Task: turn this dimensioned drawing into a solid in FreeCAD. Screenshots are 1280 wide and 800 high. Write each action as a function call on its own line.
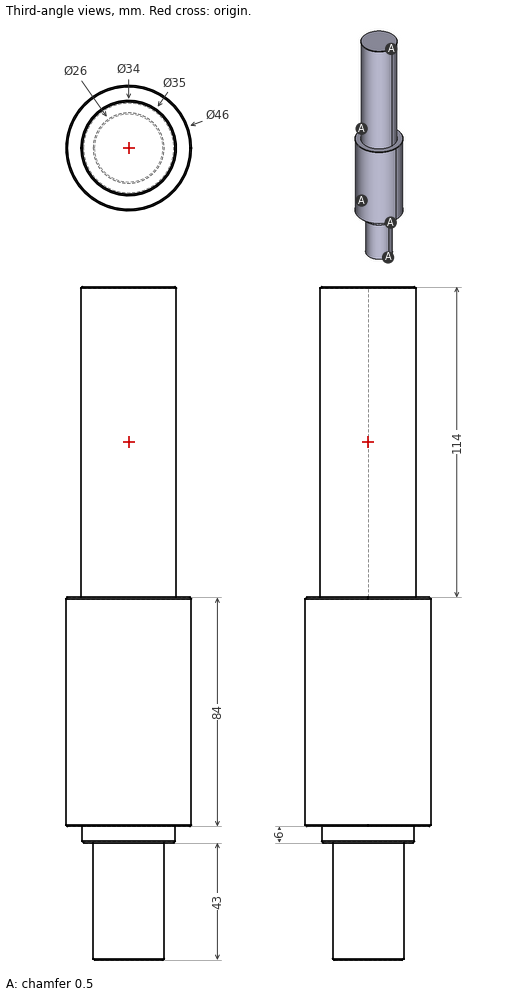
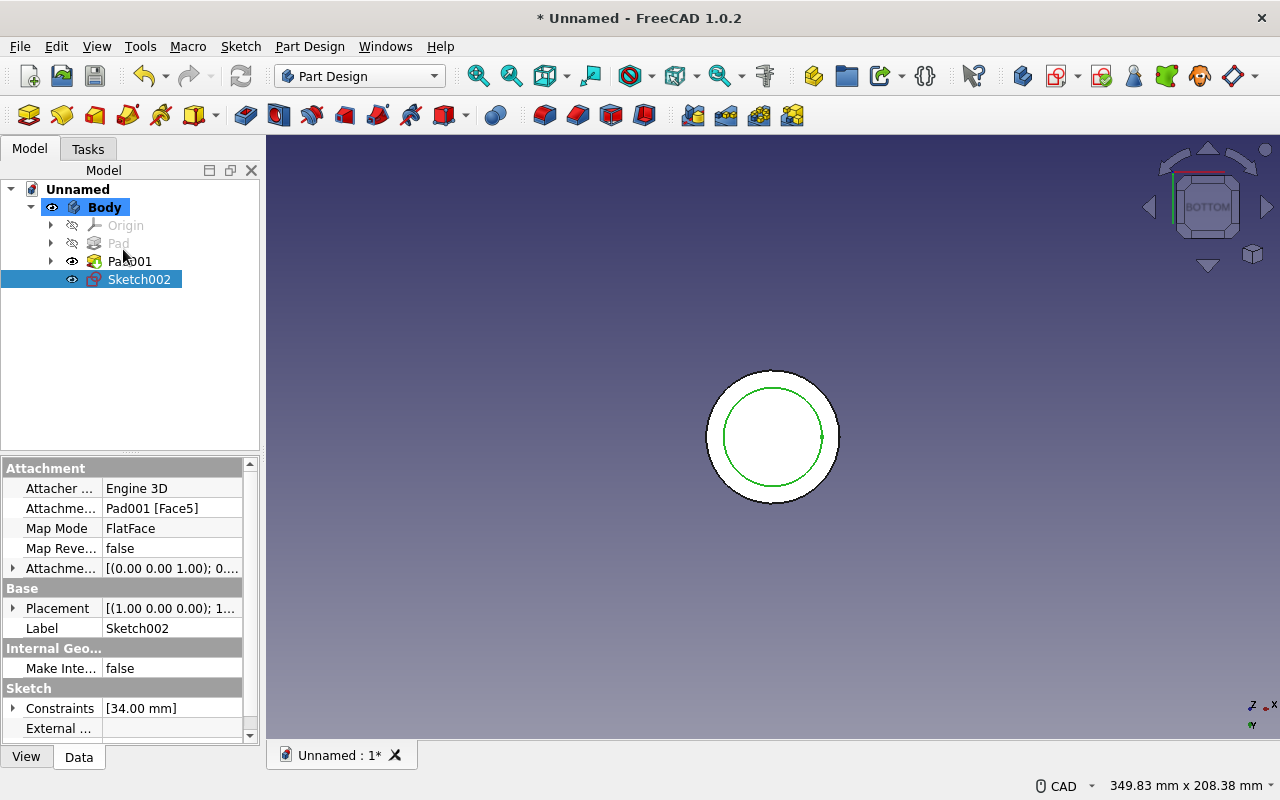
click(29, 116)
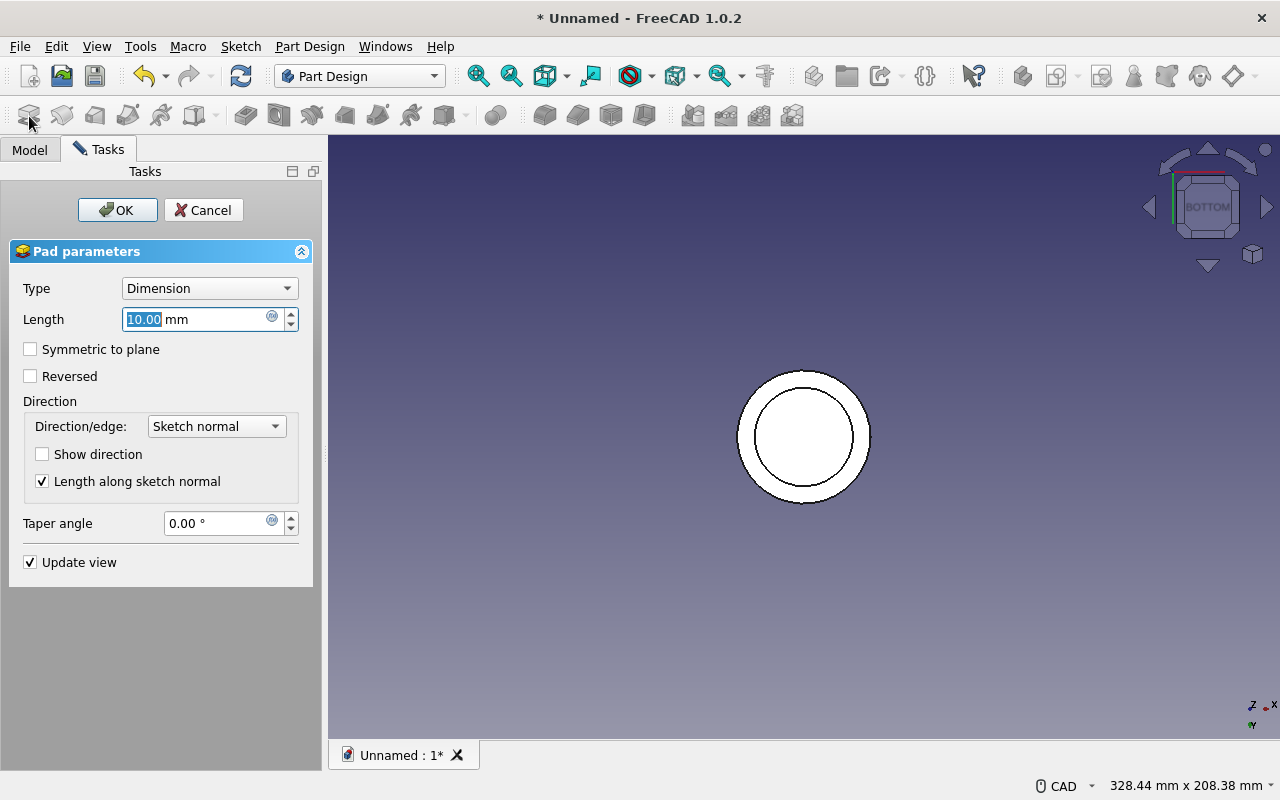
text(6)
key(Tab)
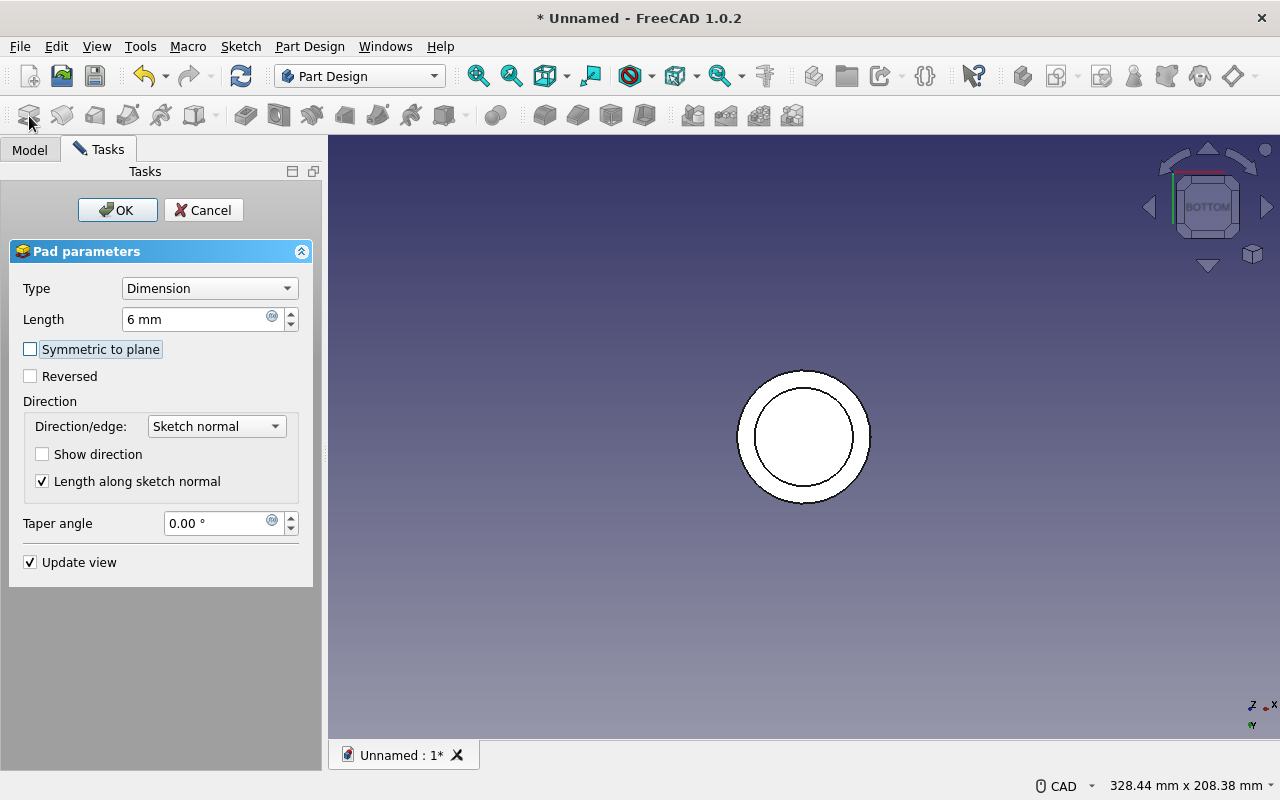
click(118, 210)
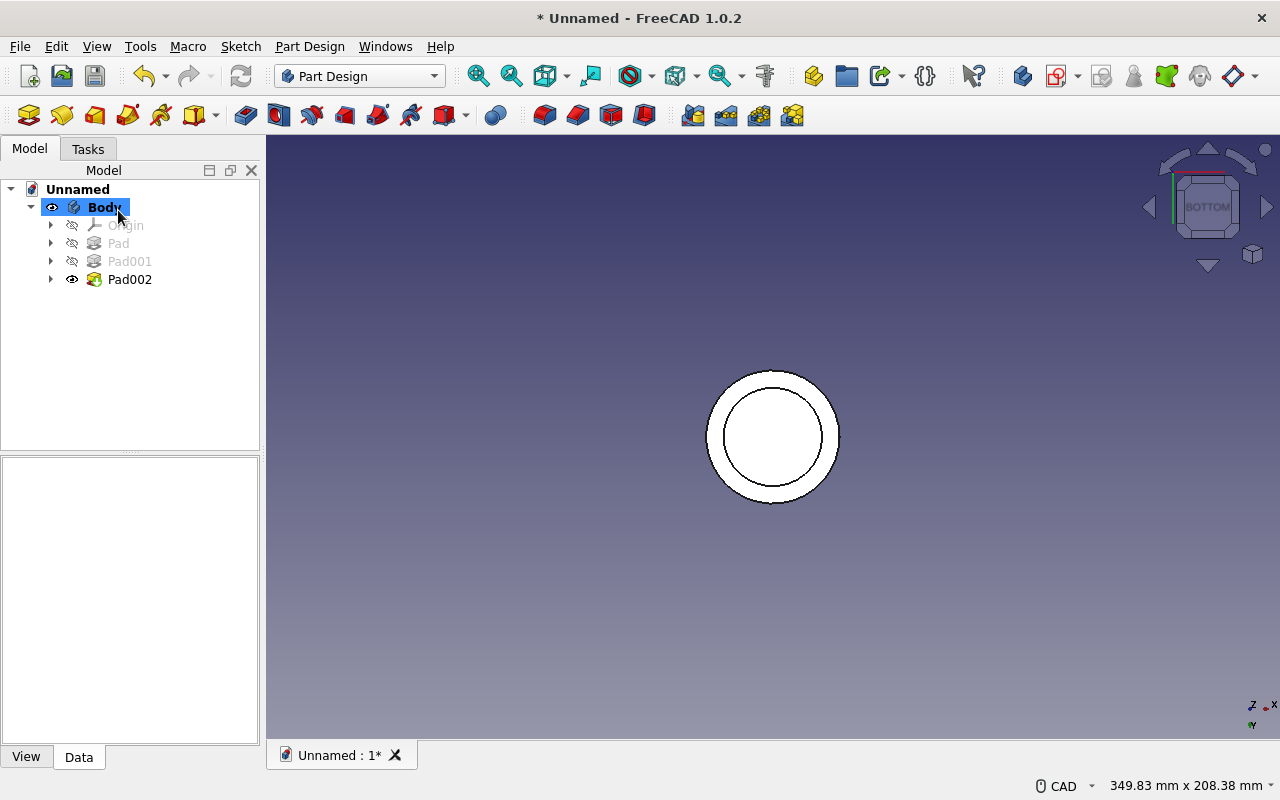
key(v)
key(f)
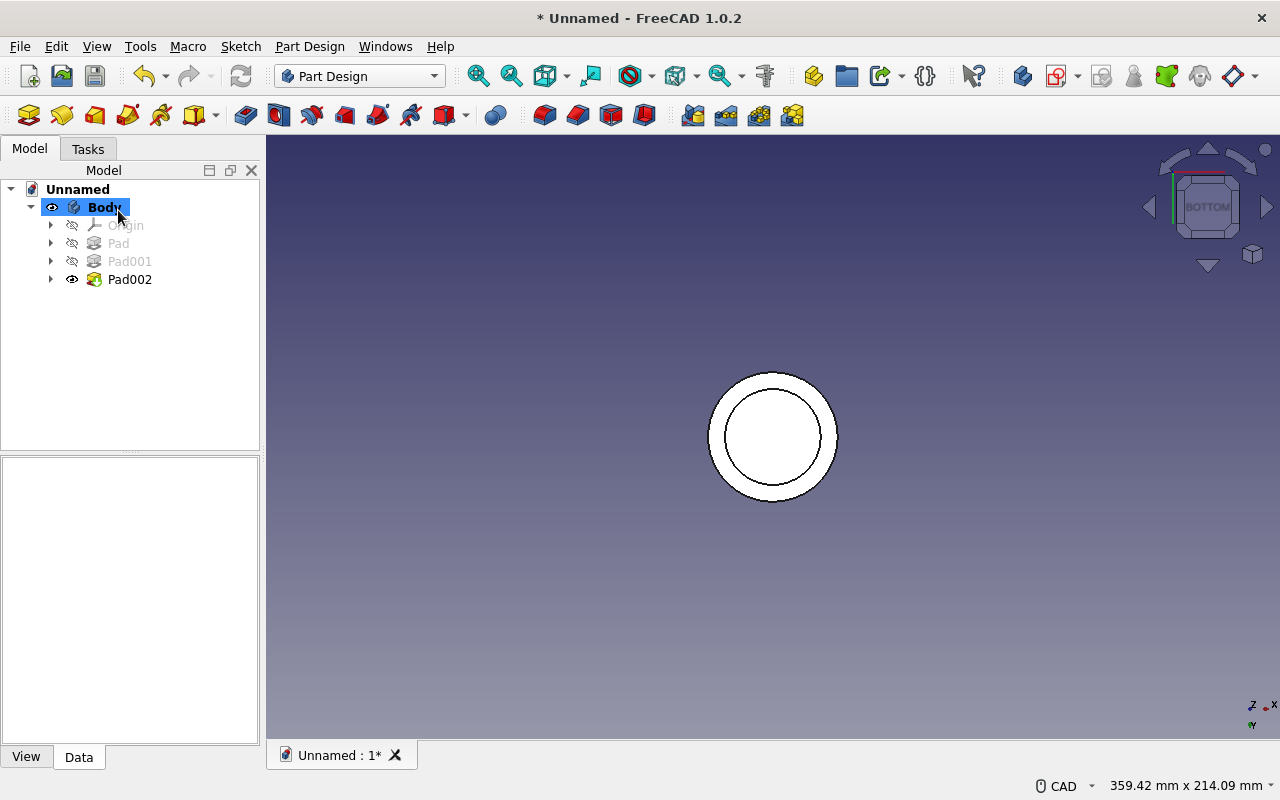
click(773, 436)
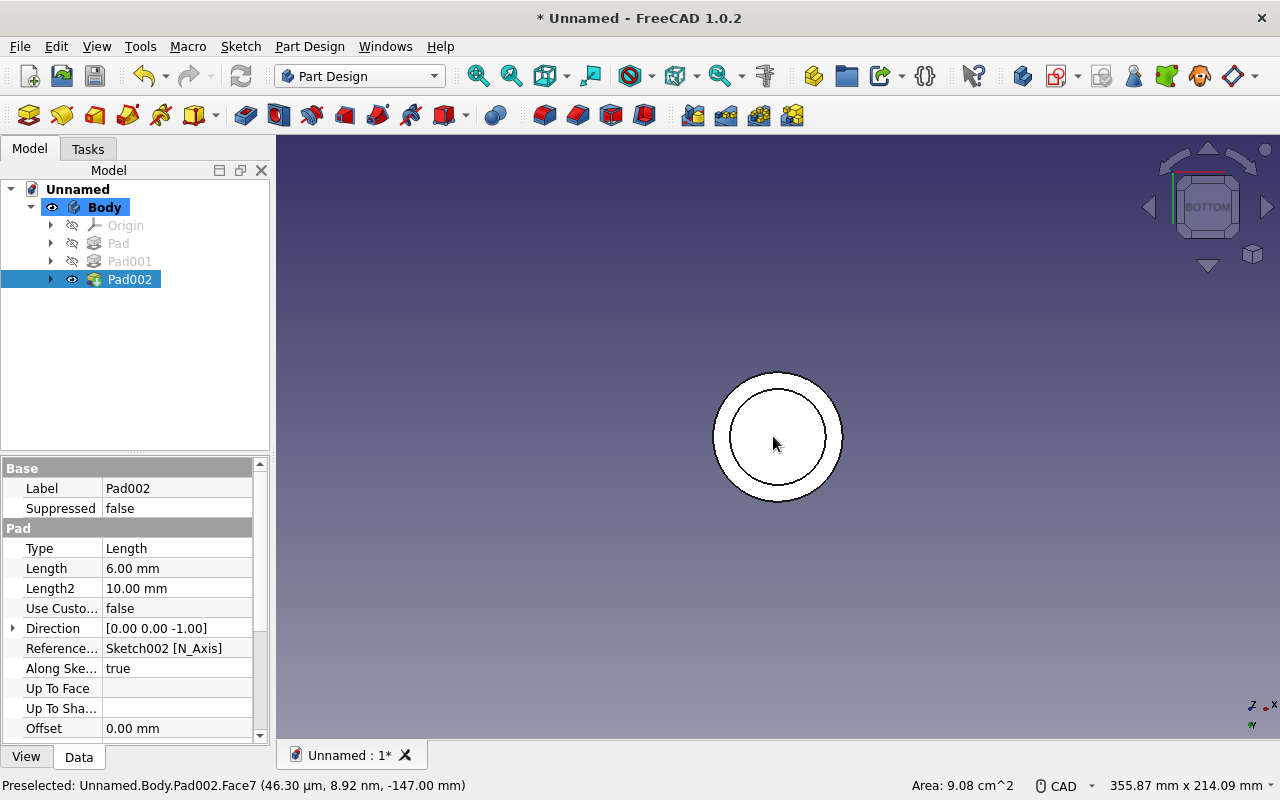
click(1056, 76)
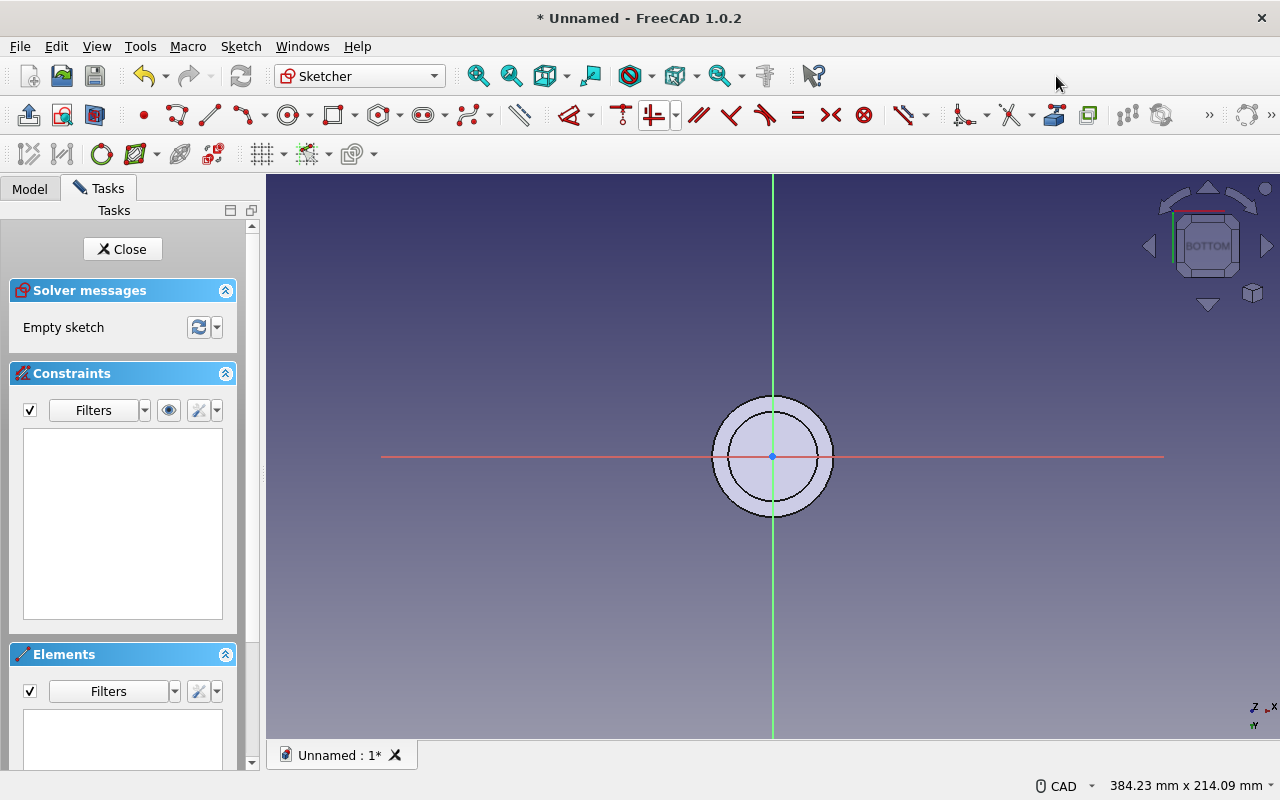
scroll(790, 456, up, 8)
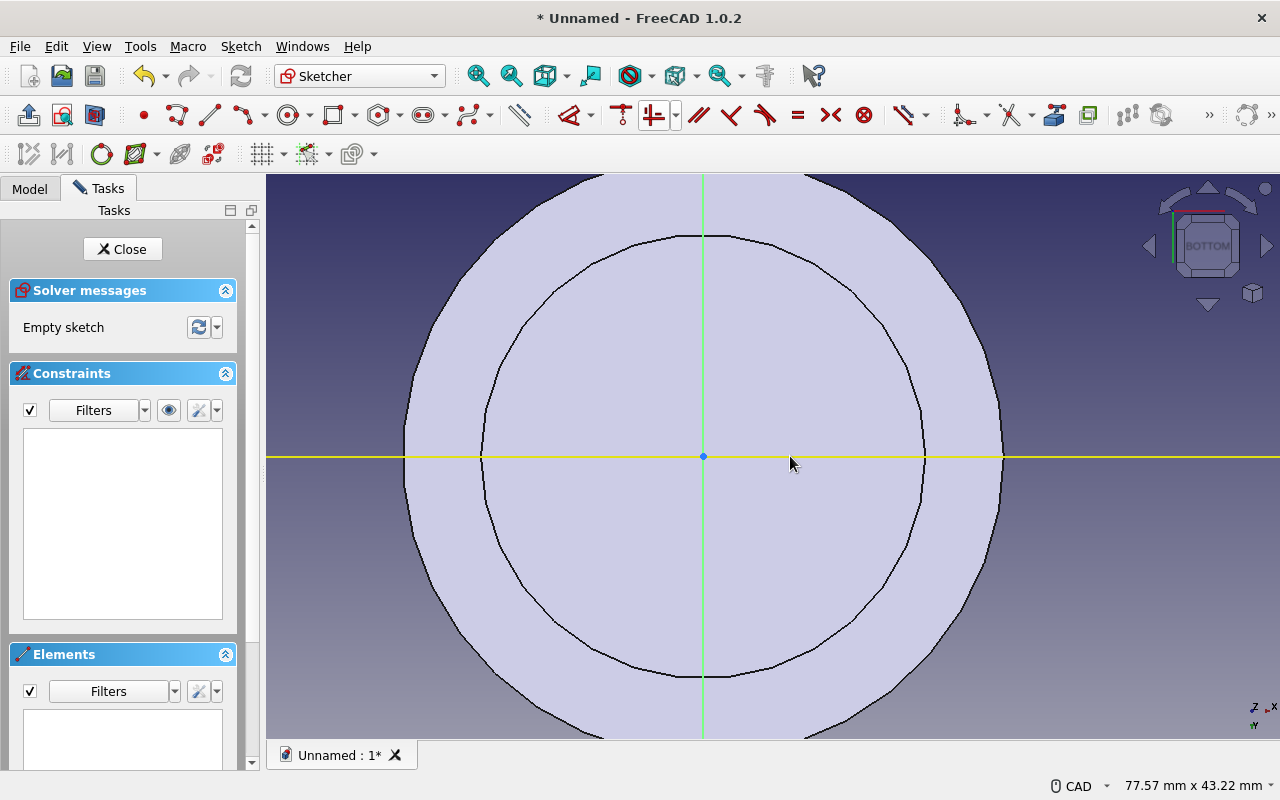
key(g)
key(c)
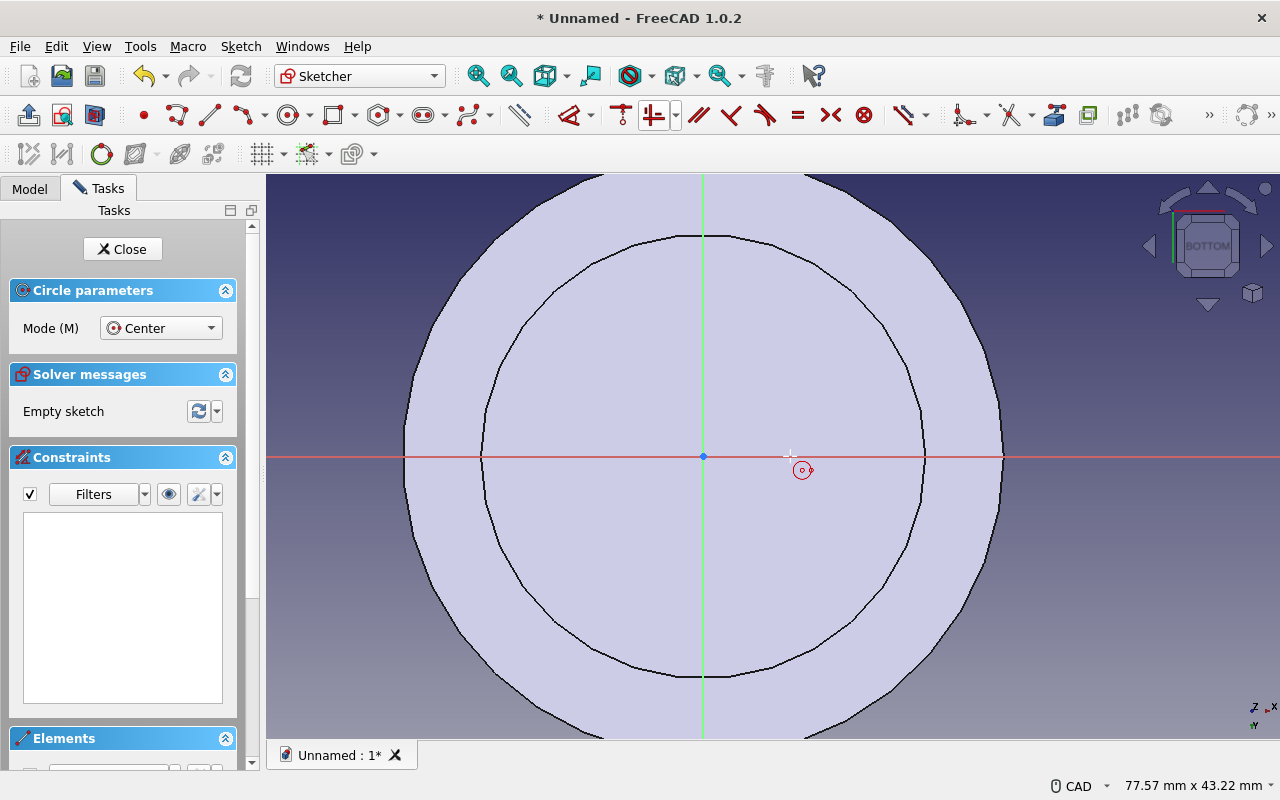
click(703, 456)
click(823, 336)
key(Escape)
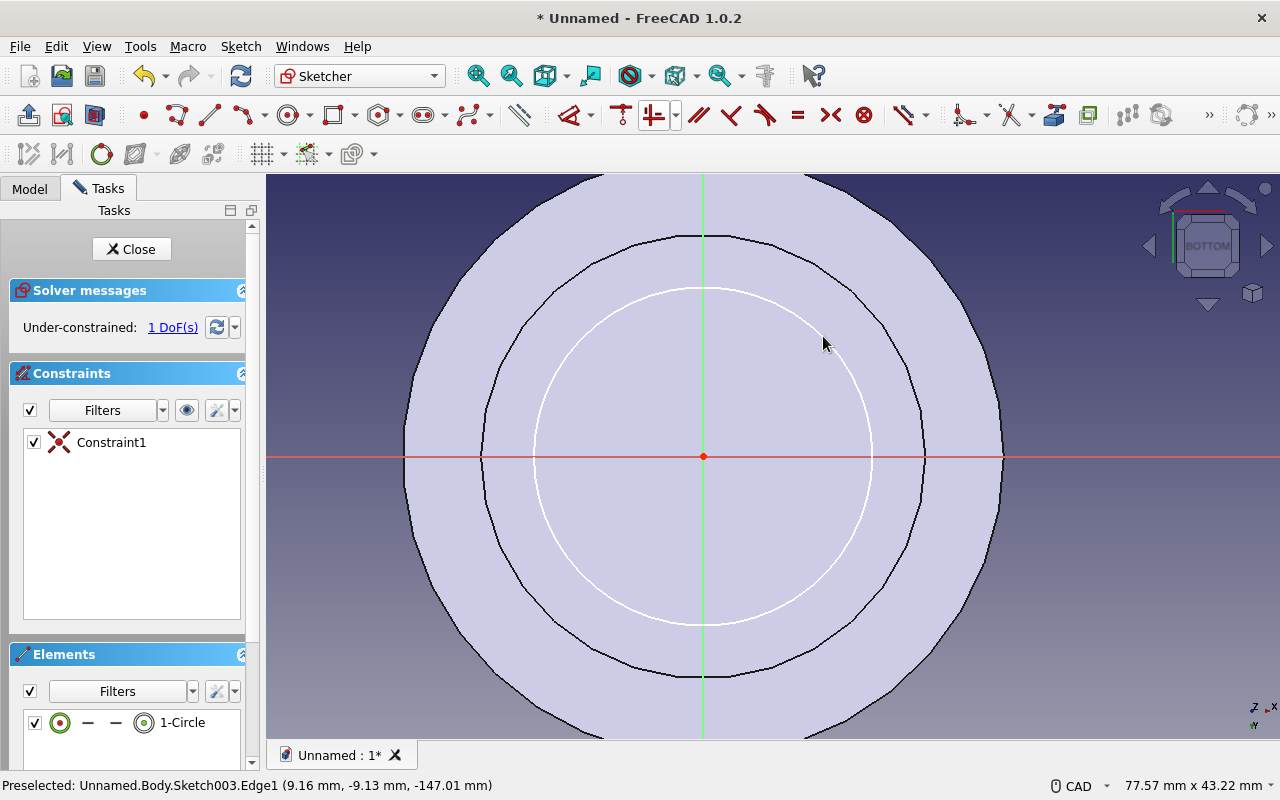
click(568, 116)